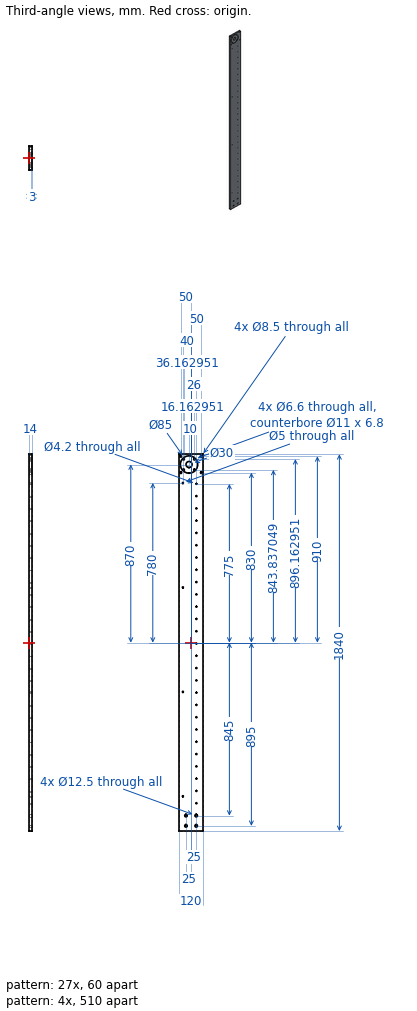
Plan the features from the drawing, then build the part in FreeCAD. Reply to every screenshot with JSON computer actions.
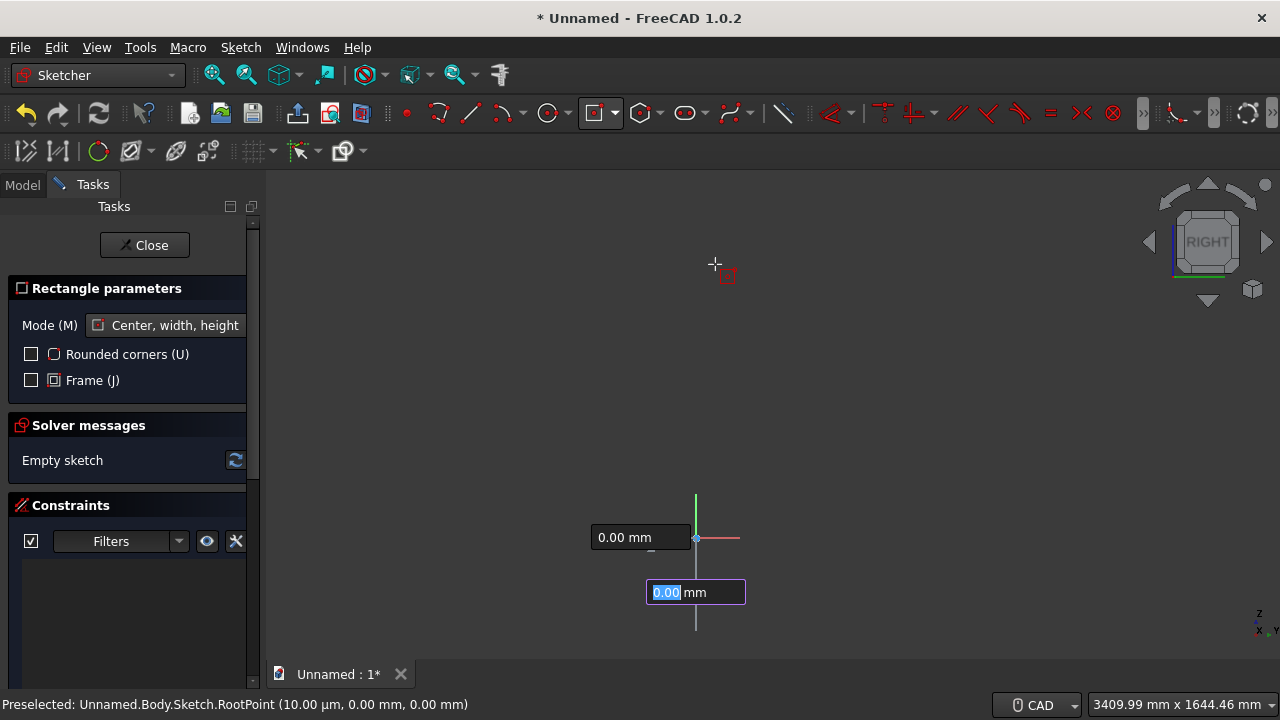
{"action": "left_click", "coordinate": [714, 264]}
{"action": "key", "text": "Escape"}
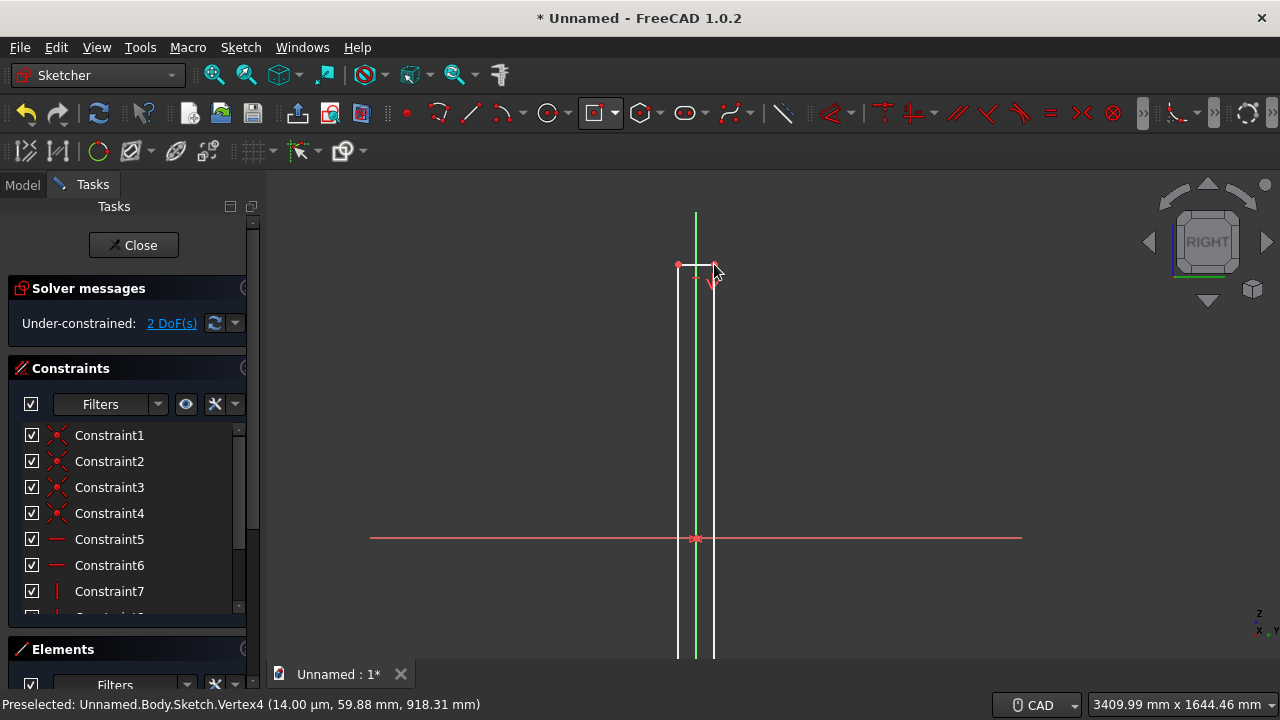
{"action": "key", "text": "d"}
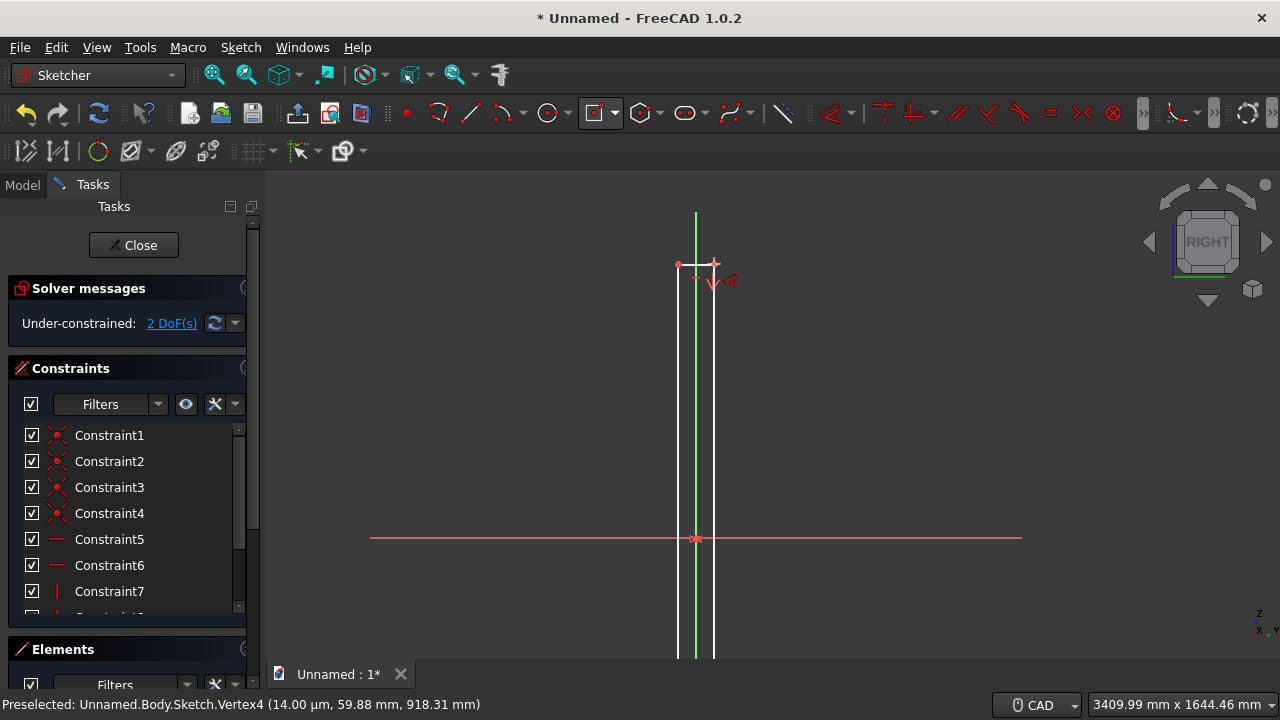
{"action": "scroll", "coordinate": [715, 264], "scroll_direction": "down", "scroll_amount": 3}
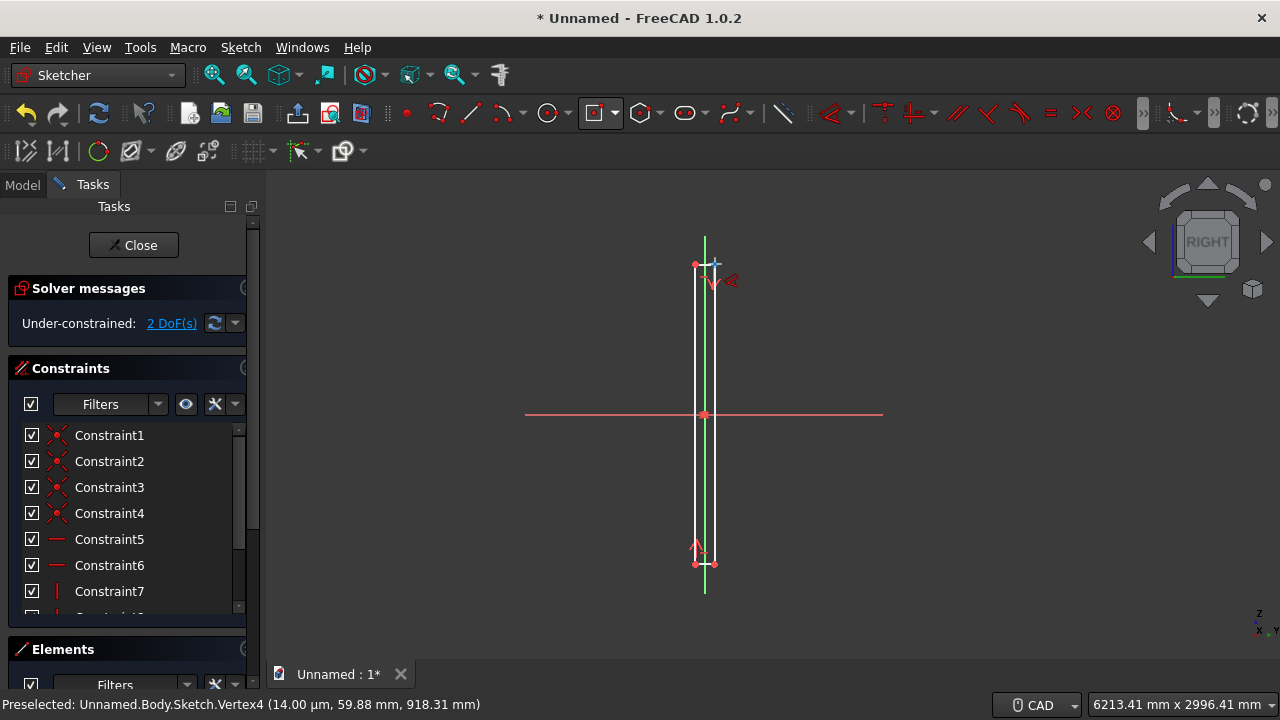
{"action": "scroll", "coordinate": [703, 564], "scroll_direction": "up", "scroll_amount": 4}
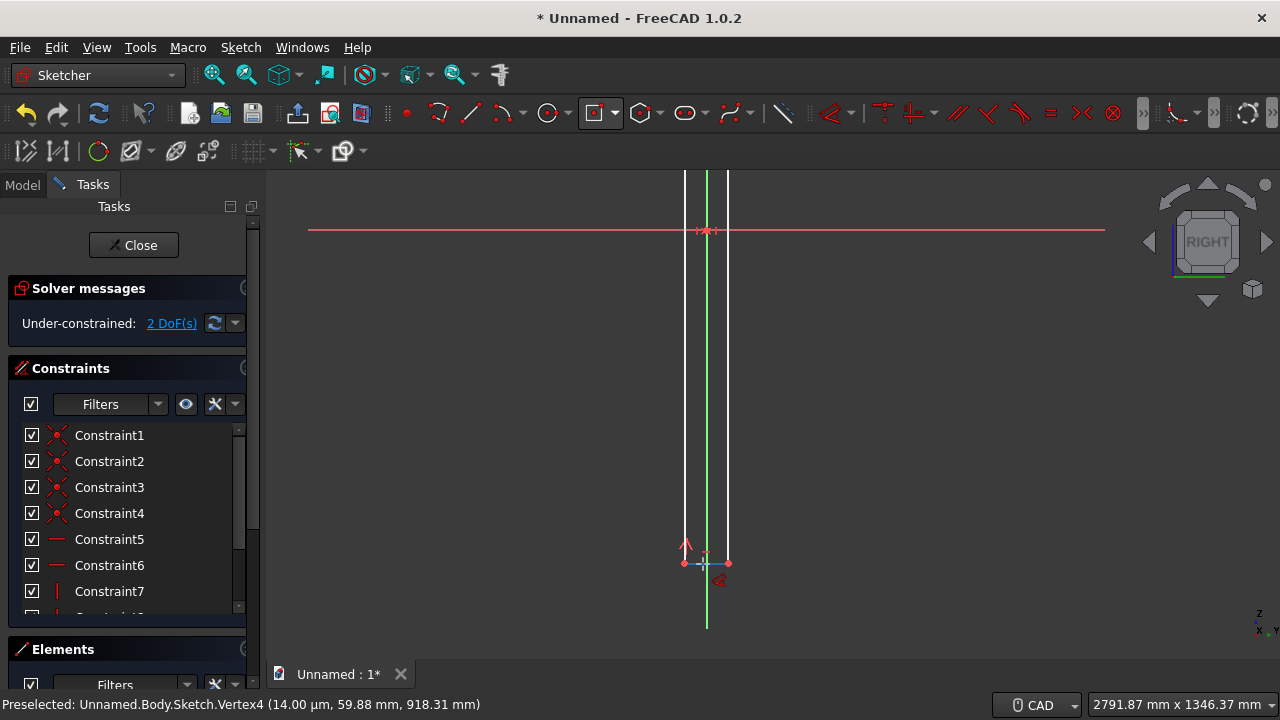
{"action": "left_click", "coordinate": [702, 564]}
{"action": "left_click", "coordinate": [691, 598]}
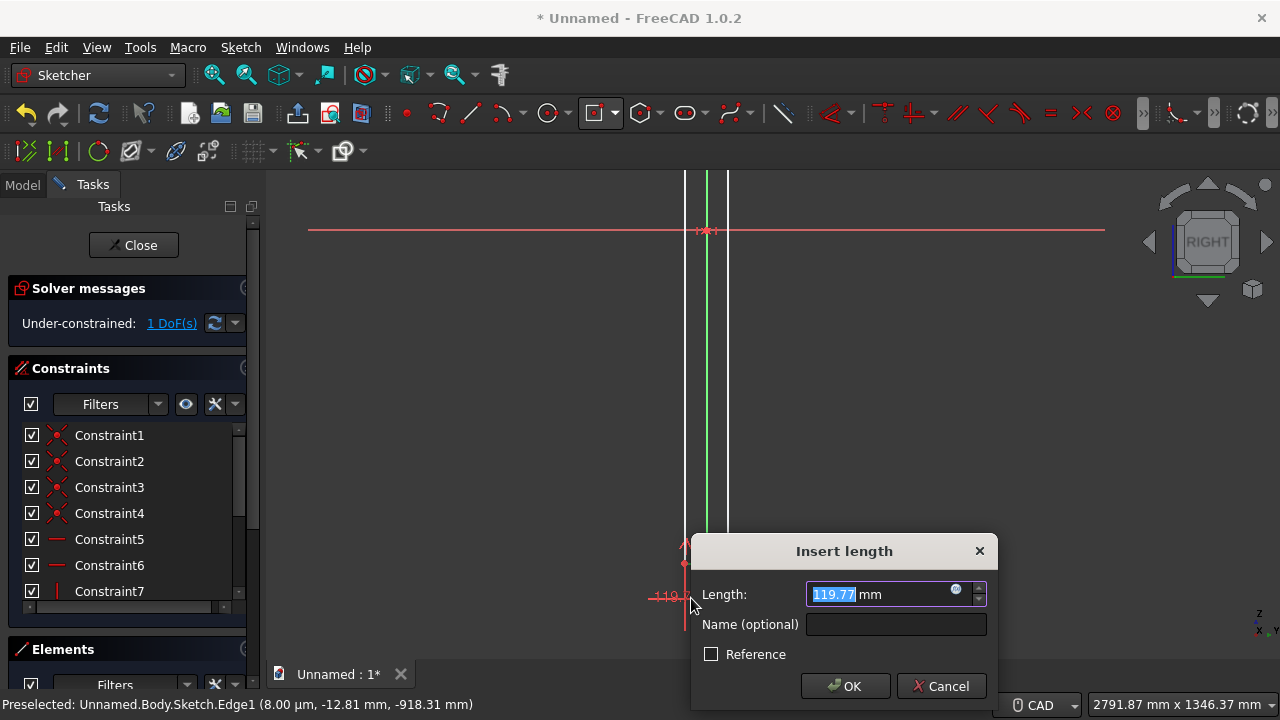
{"action": "type", "text": "120"}
{"action": "key", "text": "Return"}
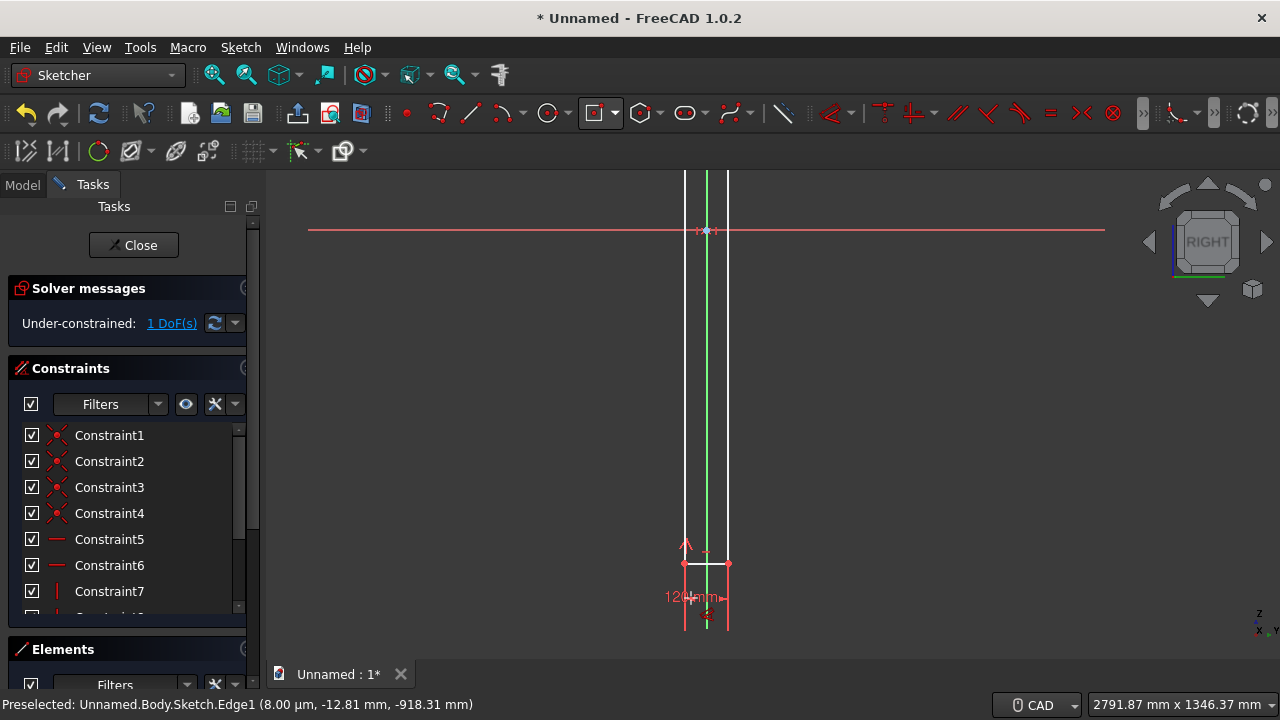
{"action": "left_click", "coordinate": [728, 364]}
{"action": "left_click", "coordinate": [762, 381]}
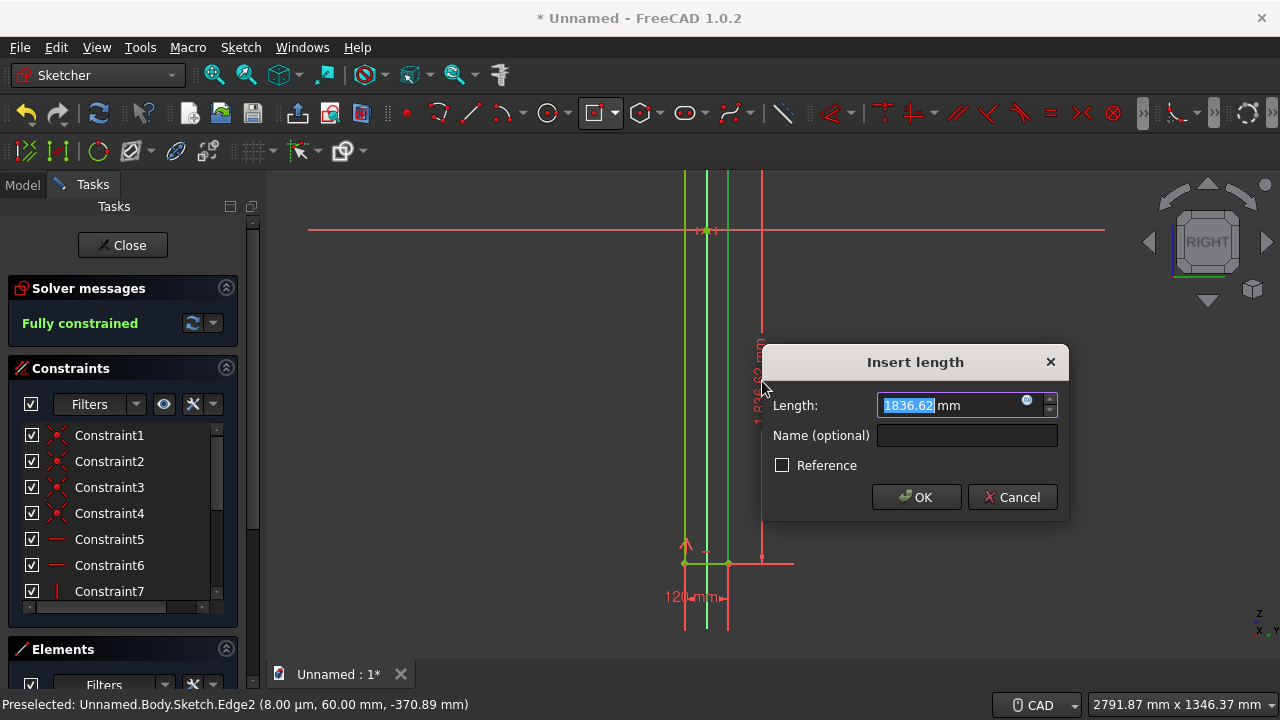
{"action": "type", "text": "1840"}
{"action": "key", "text": "Return"}
{"action": "key", "text": "Escape"}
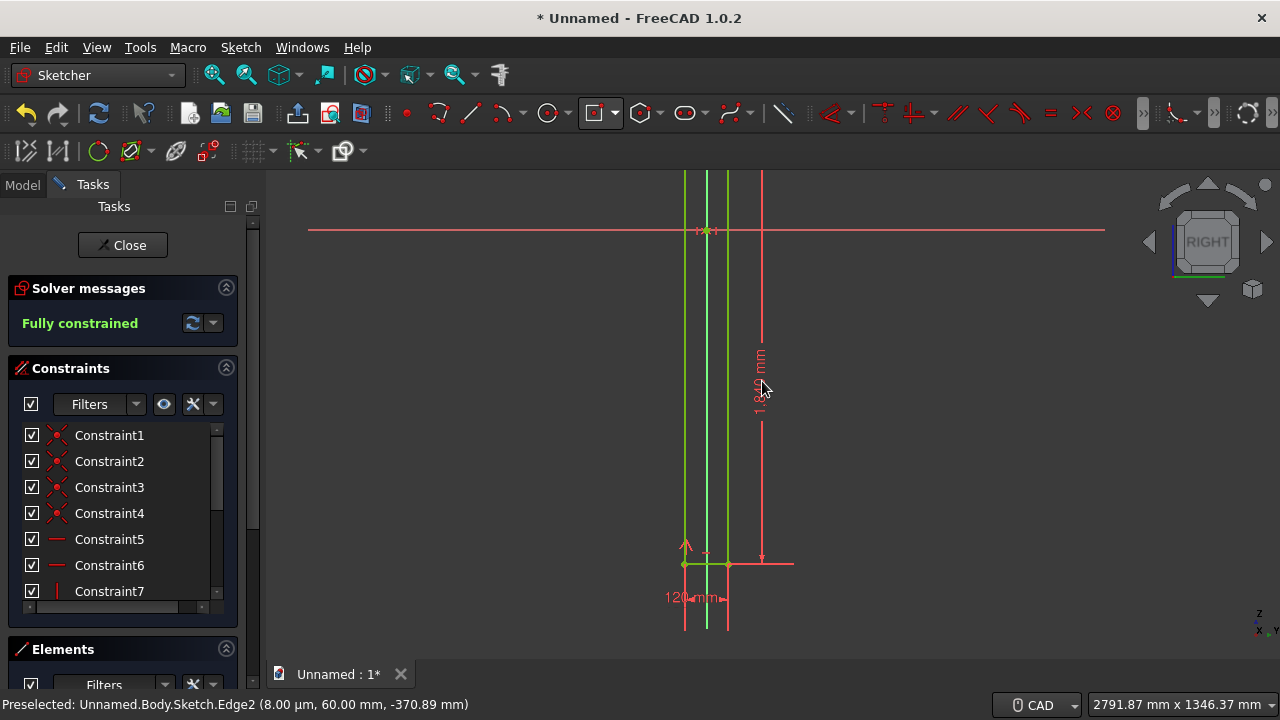
{"action": "left_click", "coordinate": [123, 245]}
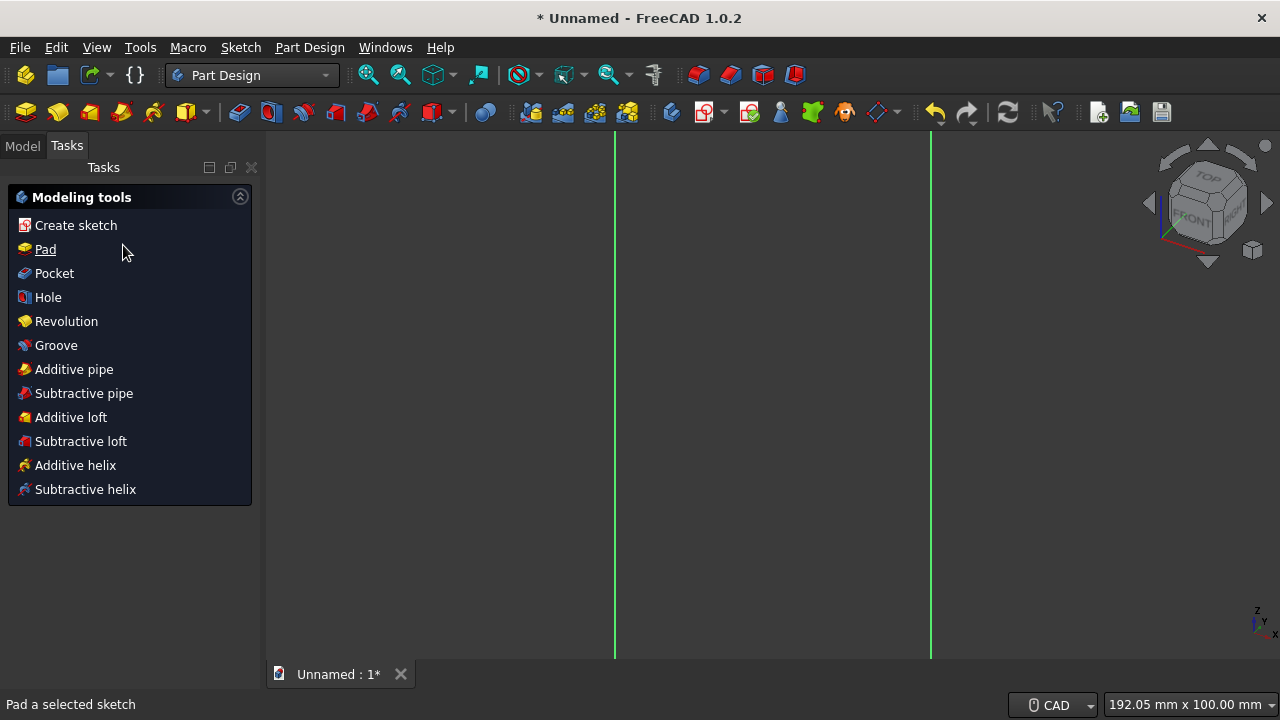
{"action": "left_click", "coordinate": [26, 112]}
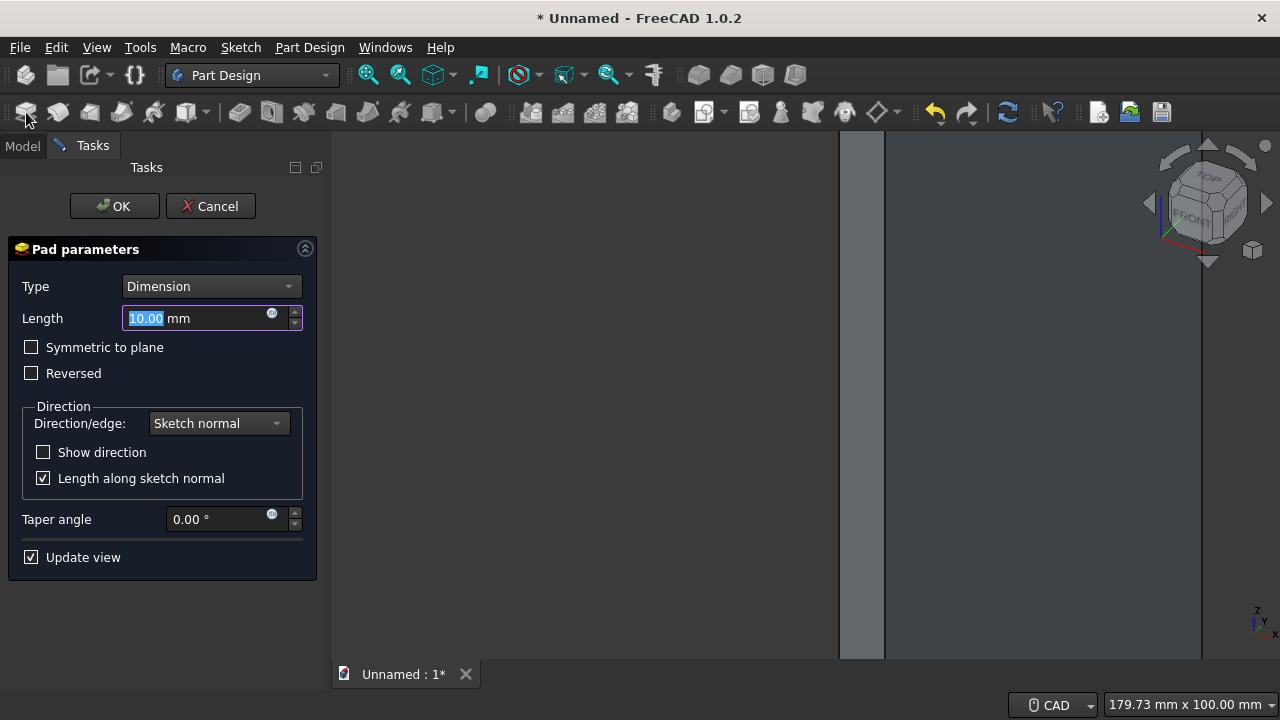
{"action": "type", "text": "14"}
{"action": "key", "text": "Tab"}